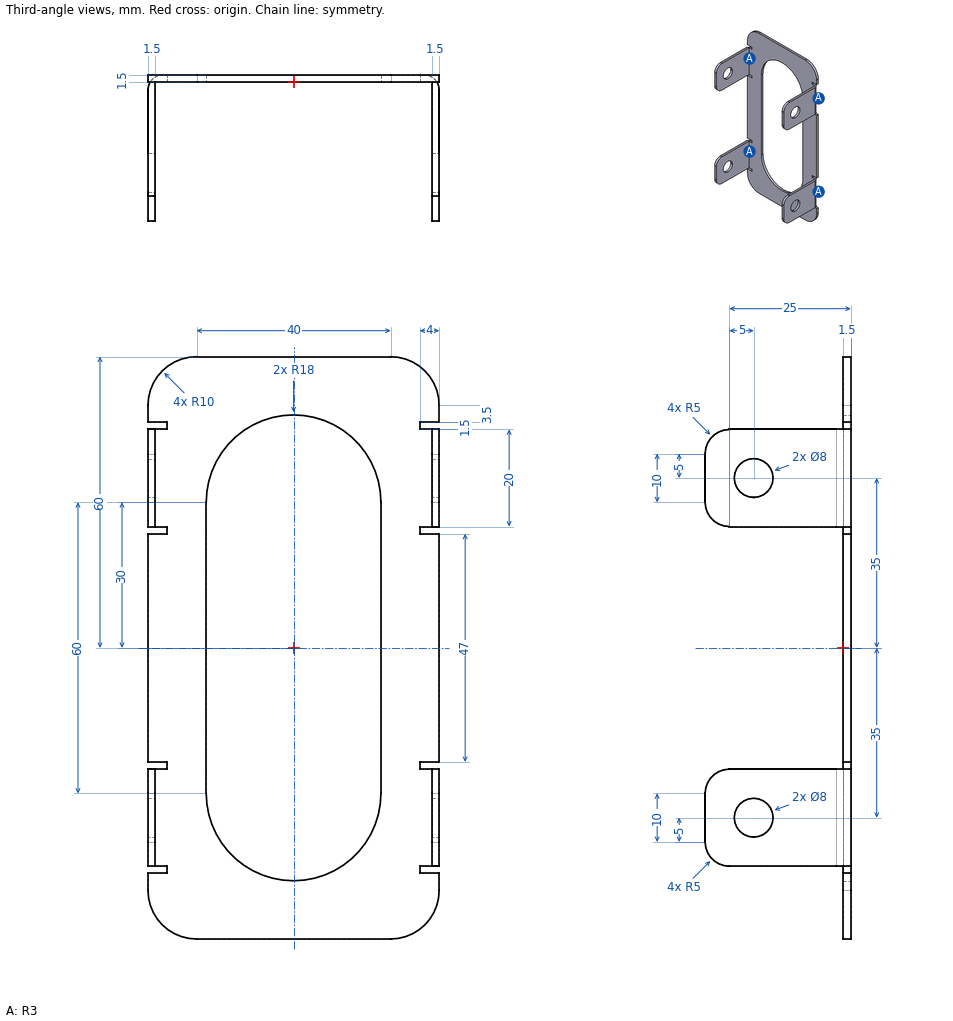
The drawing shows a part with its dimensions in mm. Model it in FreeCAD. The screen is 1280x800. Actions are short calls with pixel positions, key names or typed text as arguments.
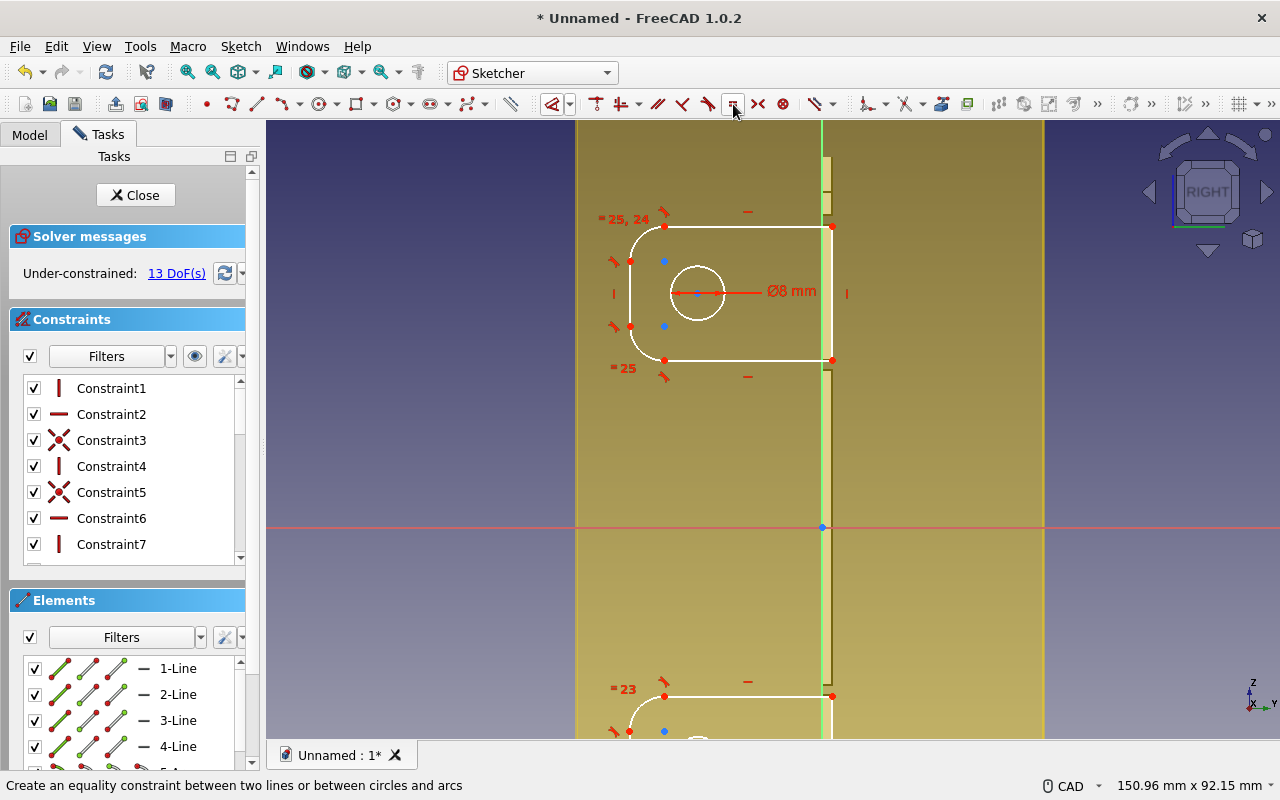
scroll(650, 230, down, 2)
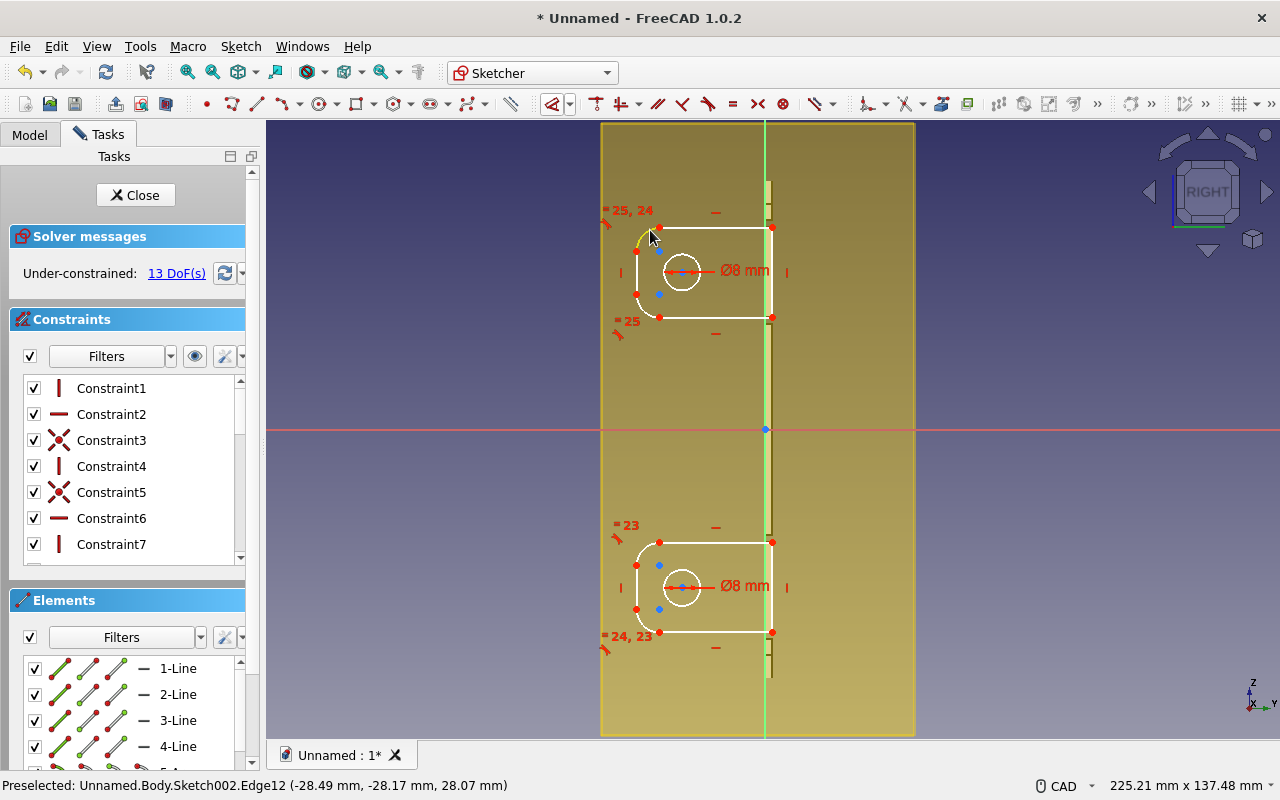
click(660, 609)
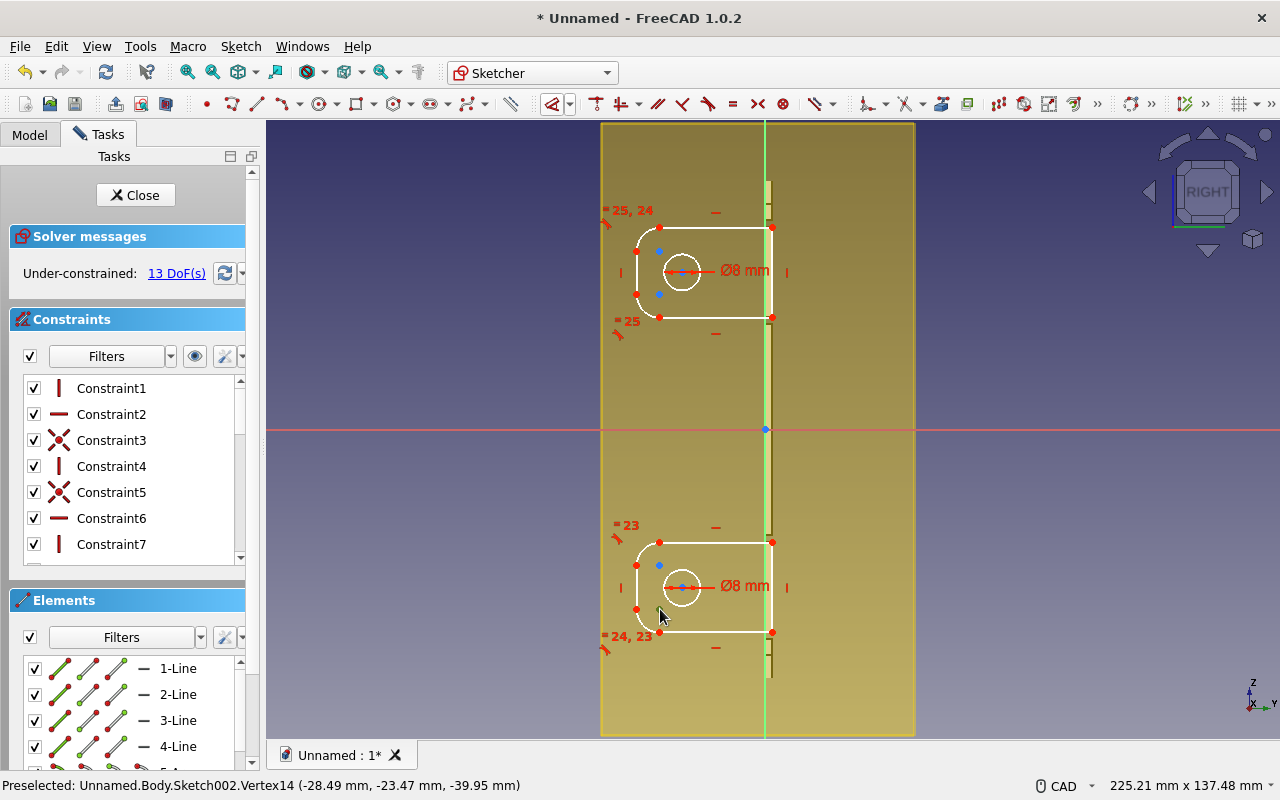
click(660, 251)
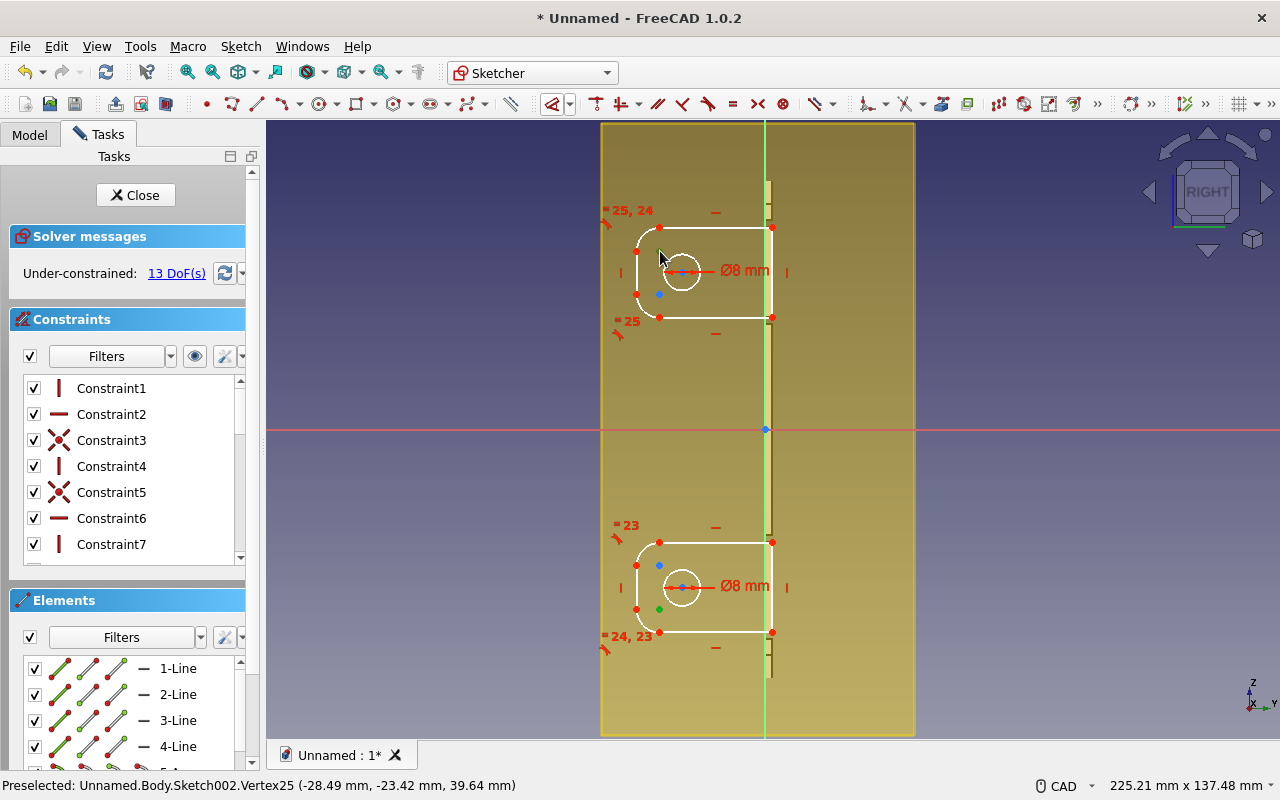
click(353, 430)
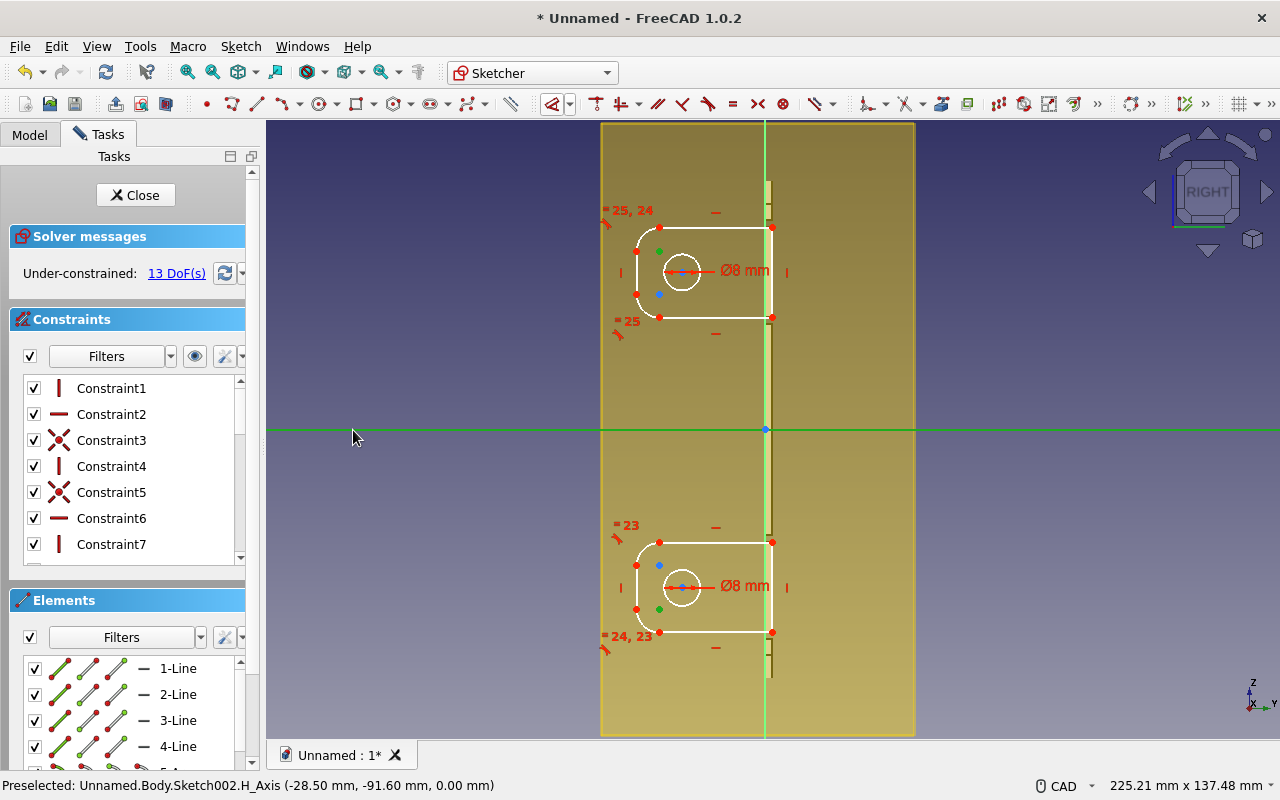
key(s)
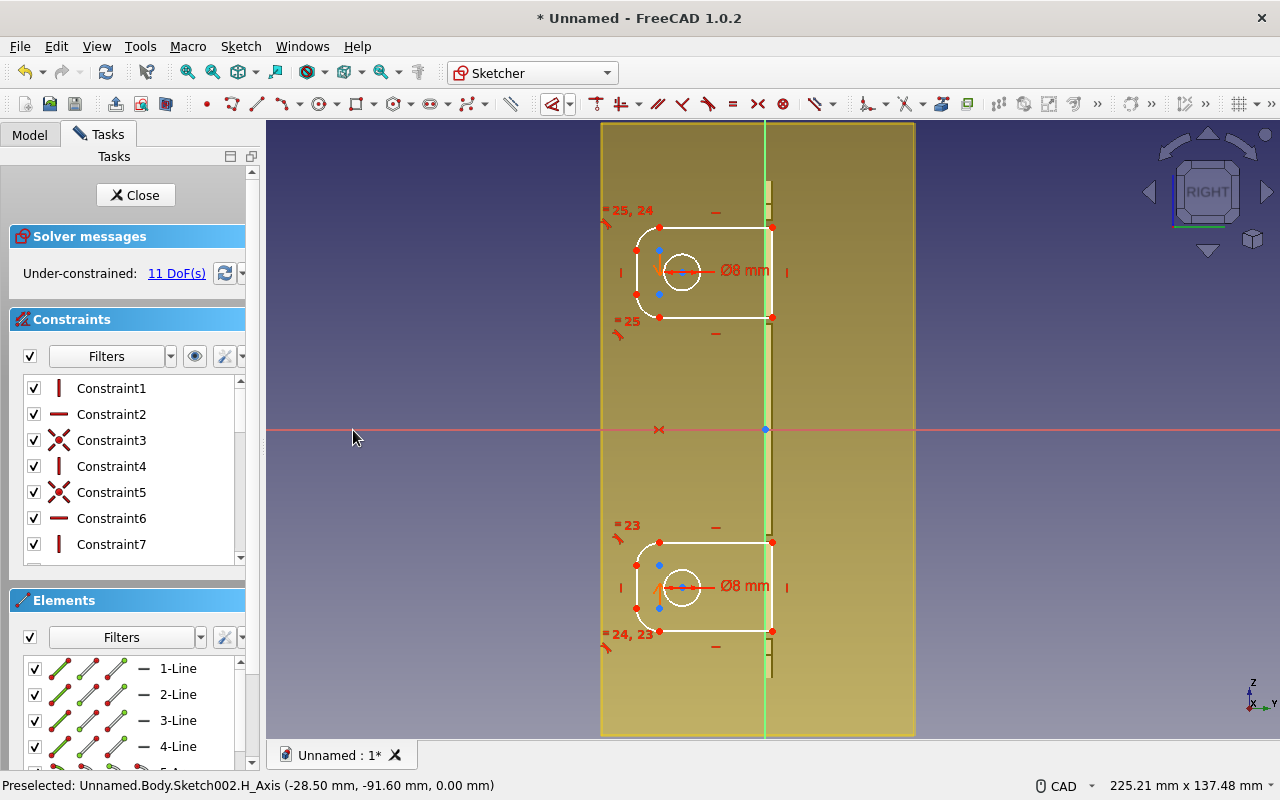
click(682, 588)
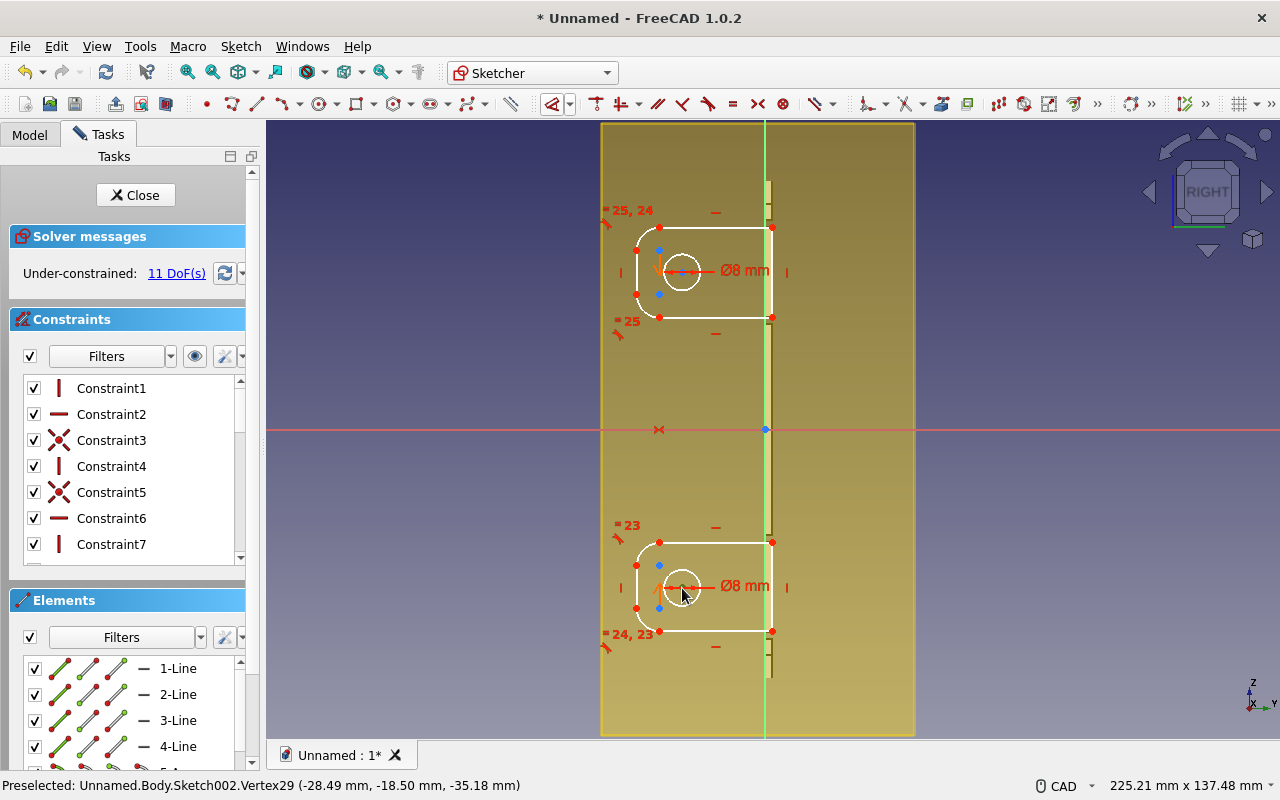
click(682, 272)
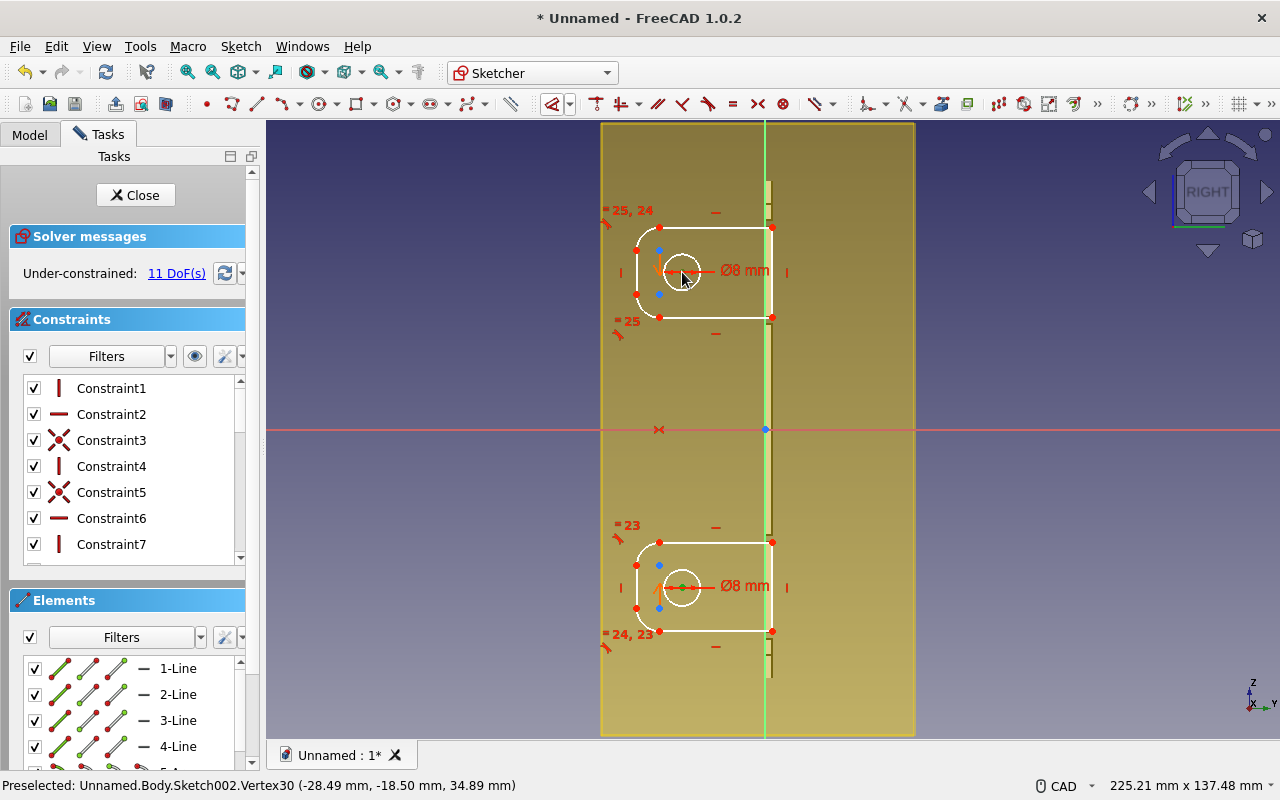
click(353, 430)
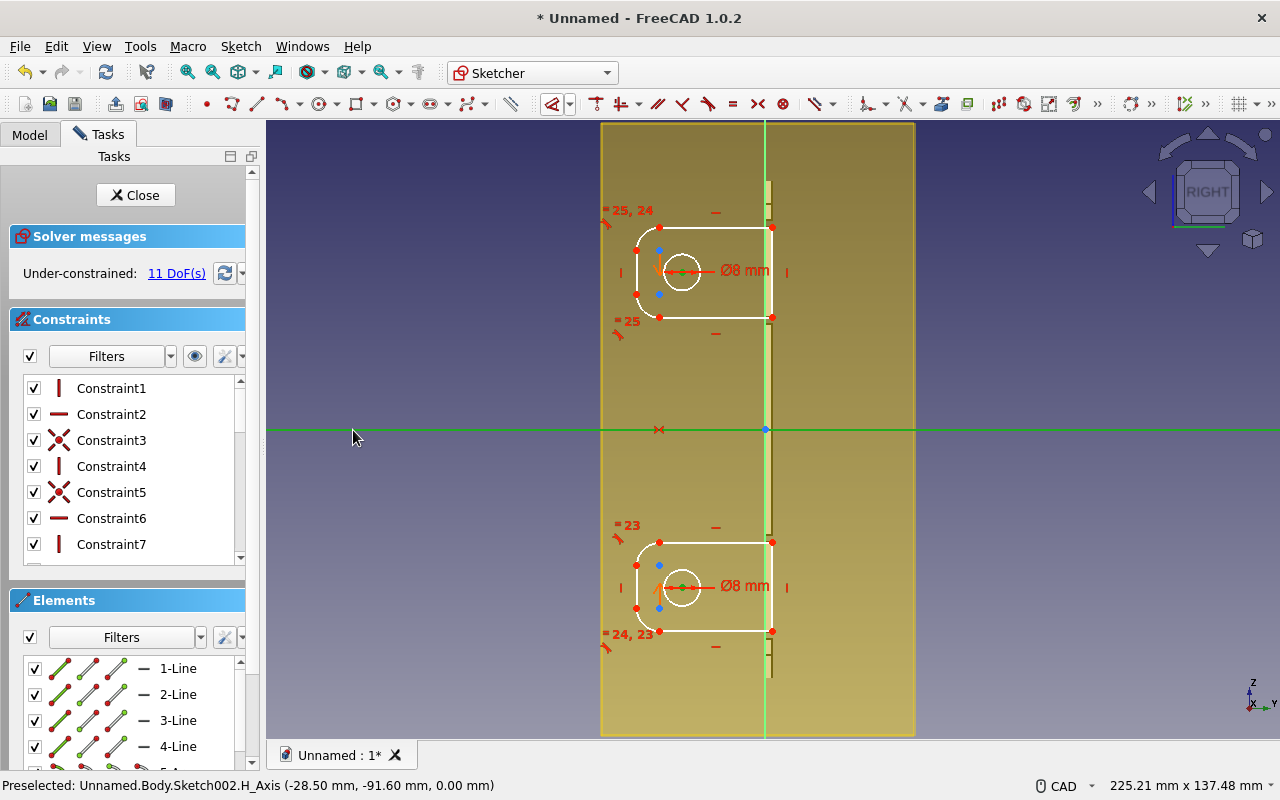
key(s)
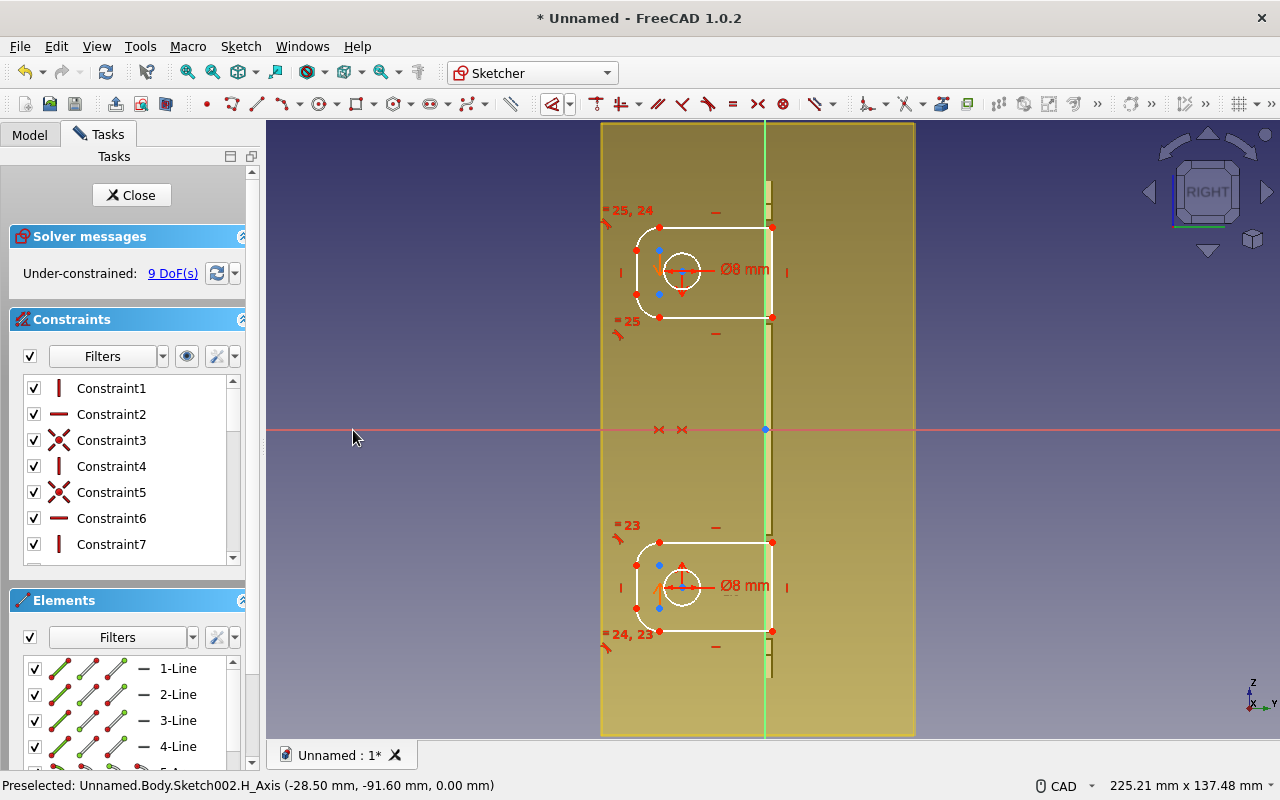
click(772, 543)